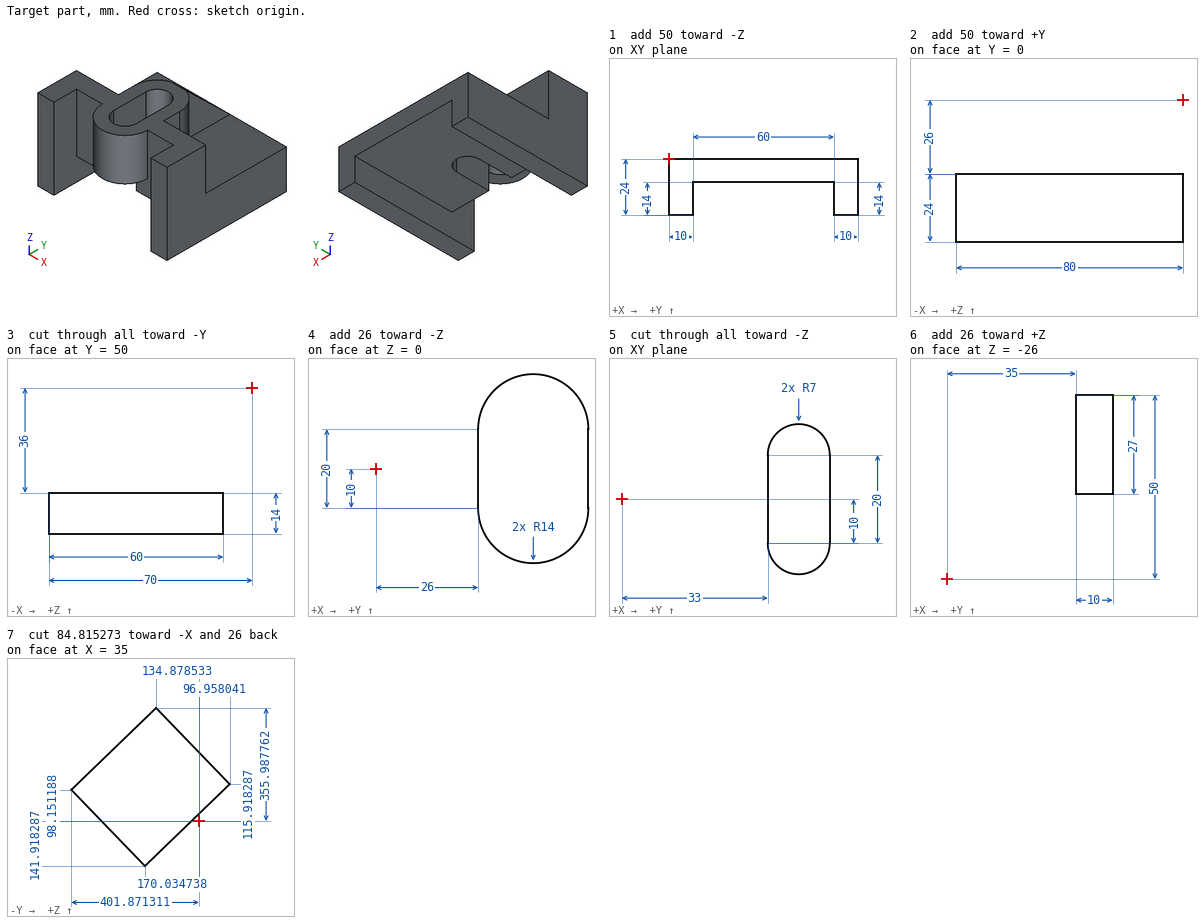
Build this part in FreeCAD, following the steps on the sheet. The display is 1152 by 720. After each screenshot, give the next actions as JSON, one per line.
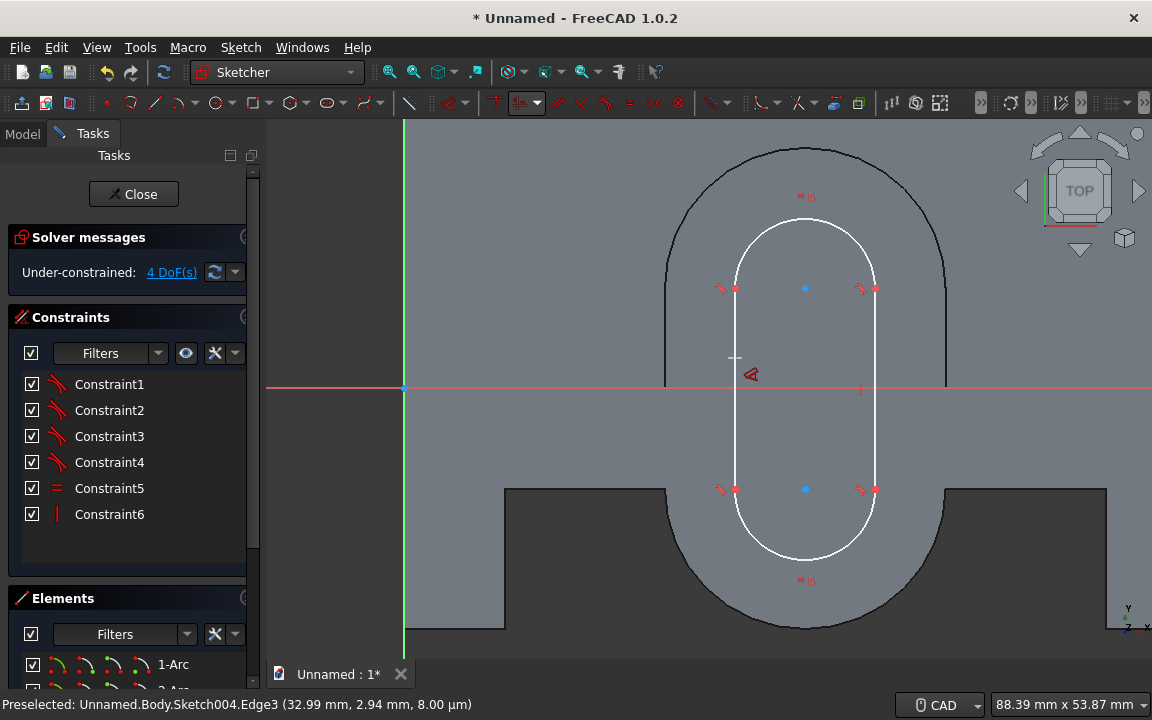
{"action": "left_click", "coordinate": [764, 547]}
{"action": "left_click", "coordinate": [745, 573]}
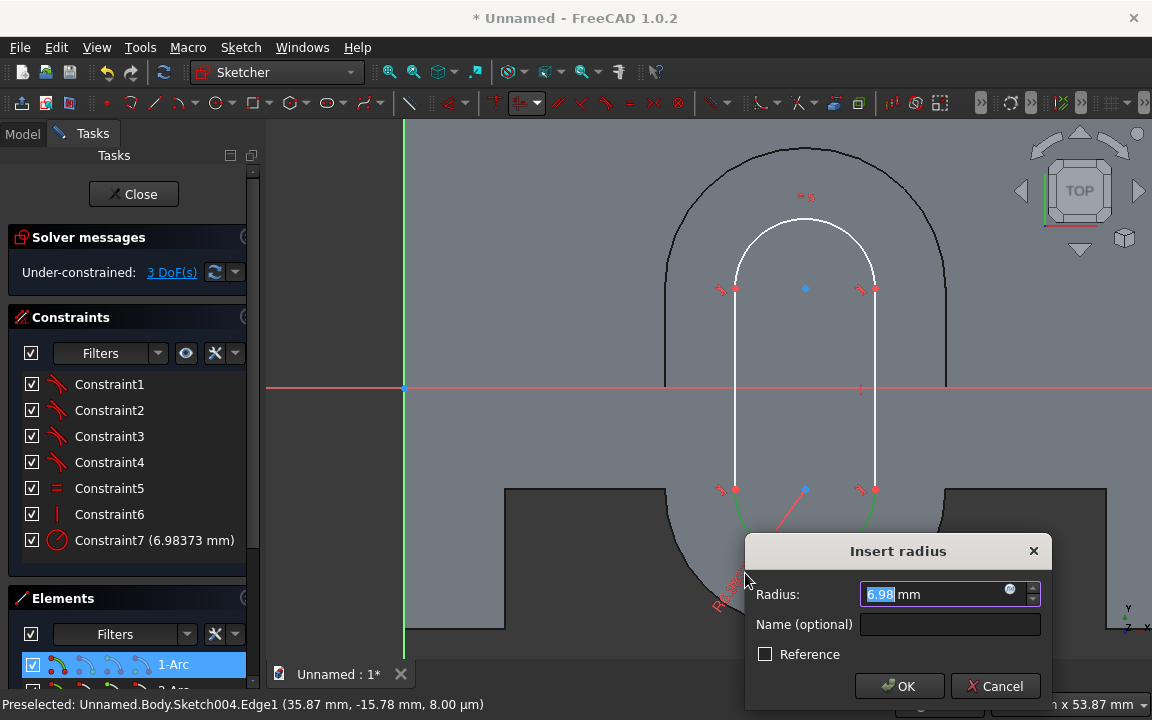
{"action": "type", "text": "7"}
{"action": "key", "text": "Return"}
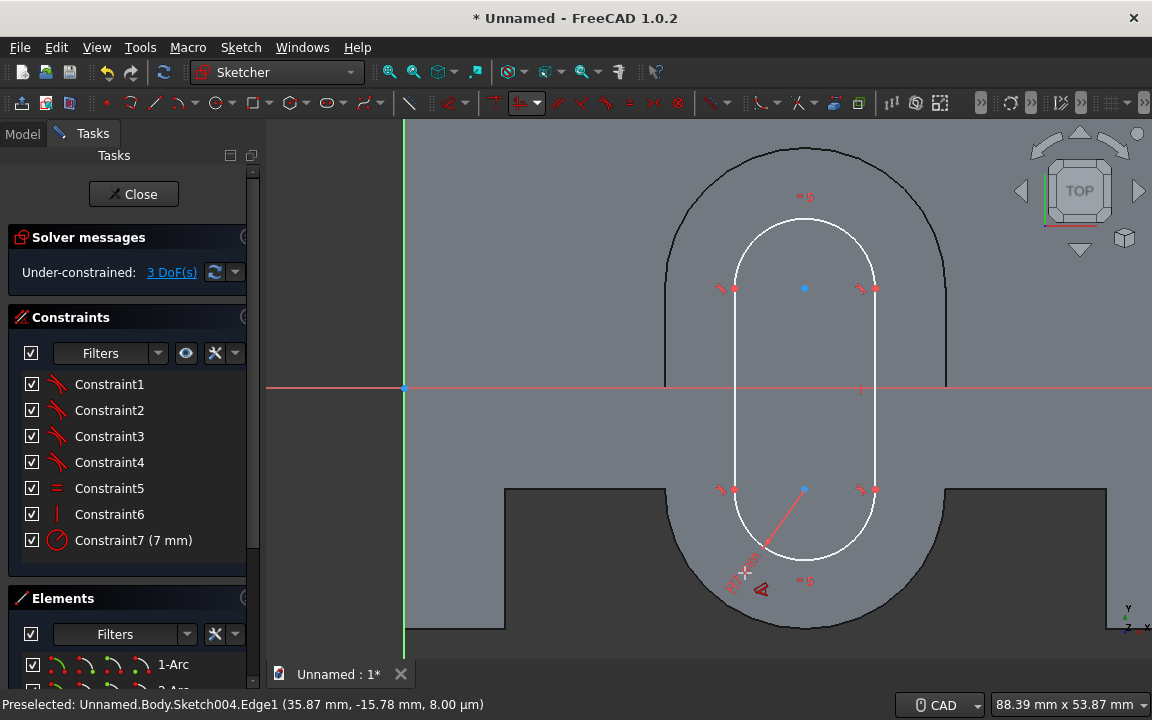
{"action": "left_click", "coordinate": [735, 430]}
{"action": "left_click", "coordinate": [769, 343]}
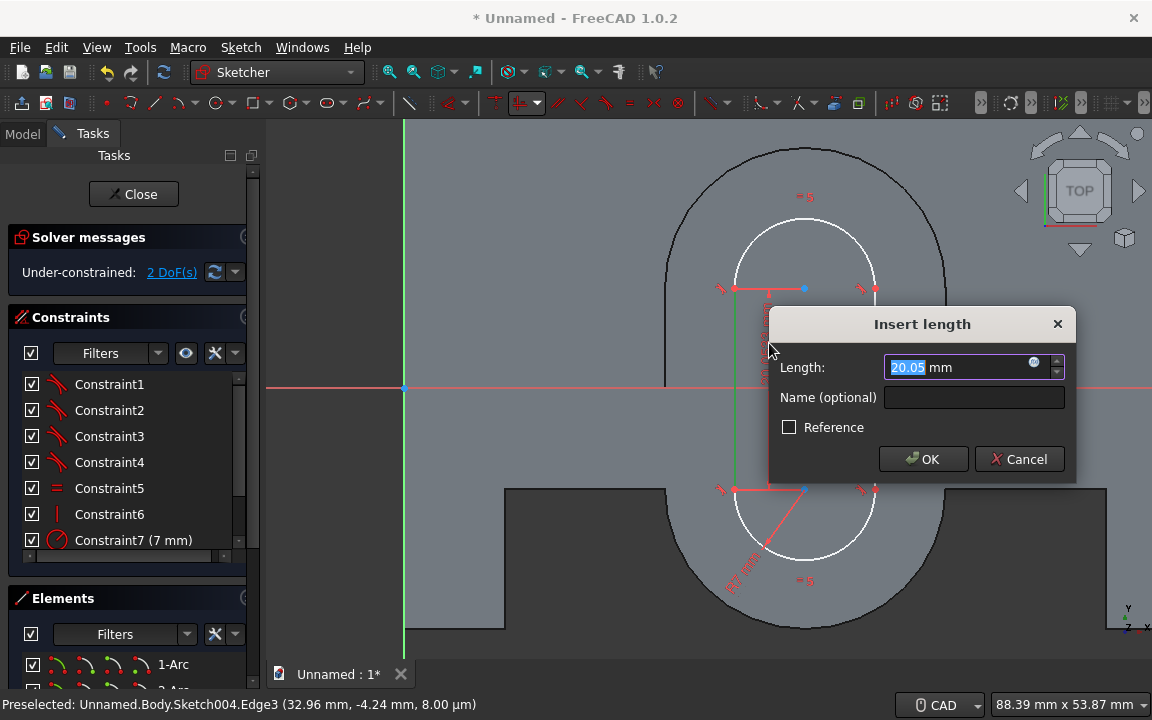
{"action": "type", "text": "20"}
{"action": "key", "text": "Return"}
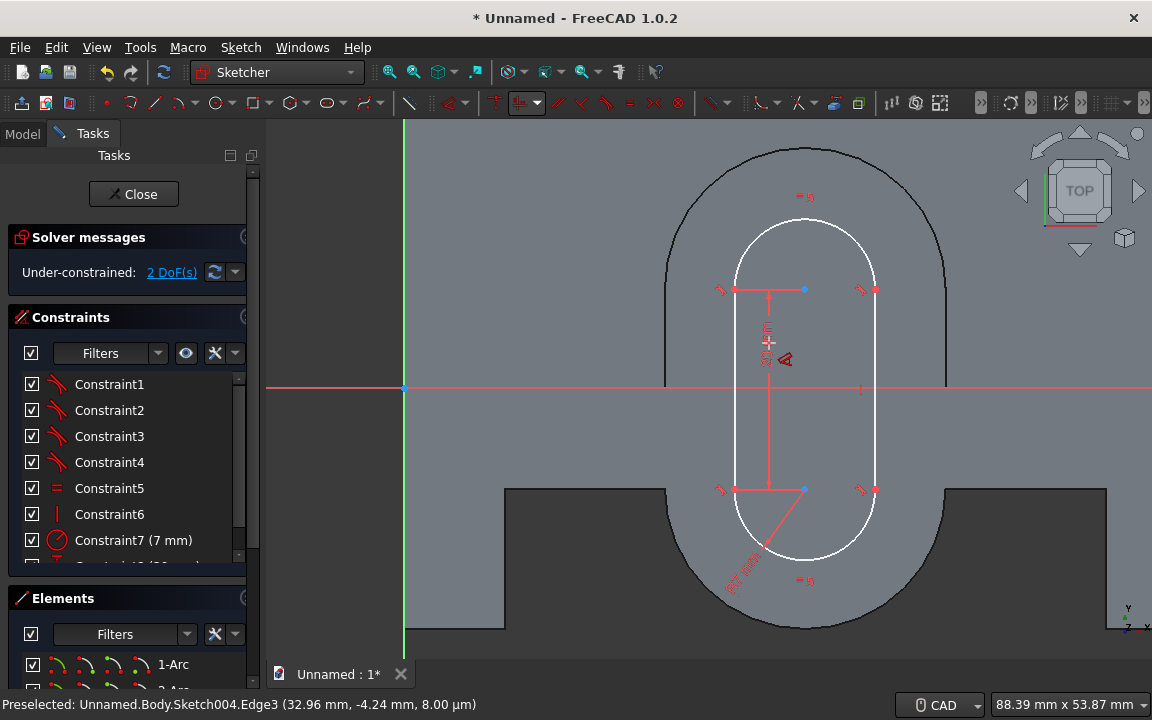
{"action": "left_click", "coordinate": [735, 490]}
{"action": "left_click", "coordinate": [569, 524]}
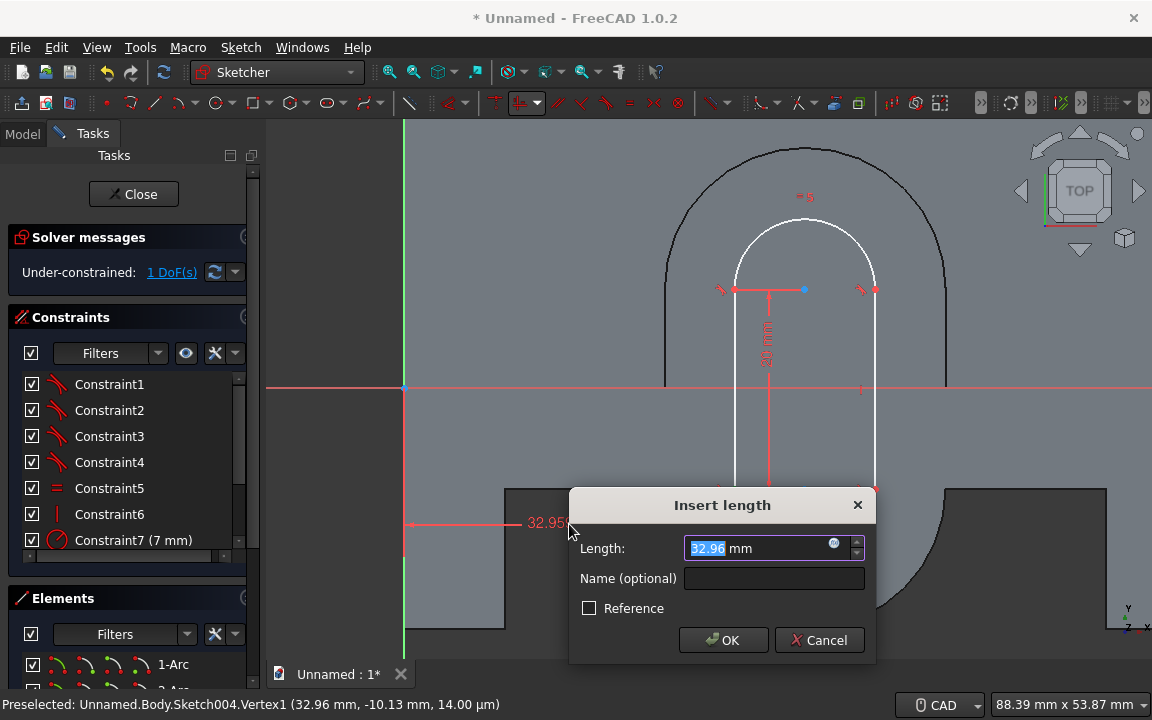
{"action": "type", "text": "33"}
{"action": "key", "text": "Return"}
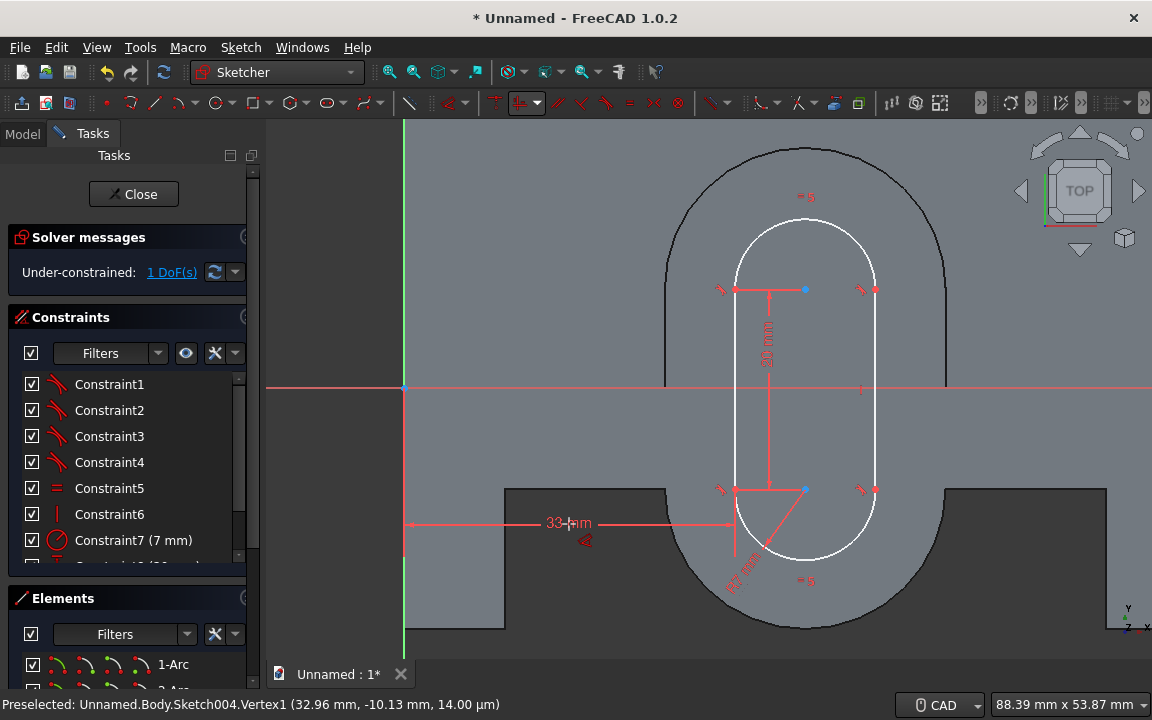
{"action": "left_click", "coordinate": [735, 490]}
{"action": "left_click", "coordinate": [370, 439]}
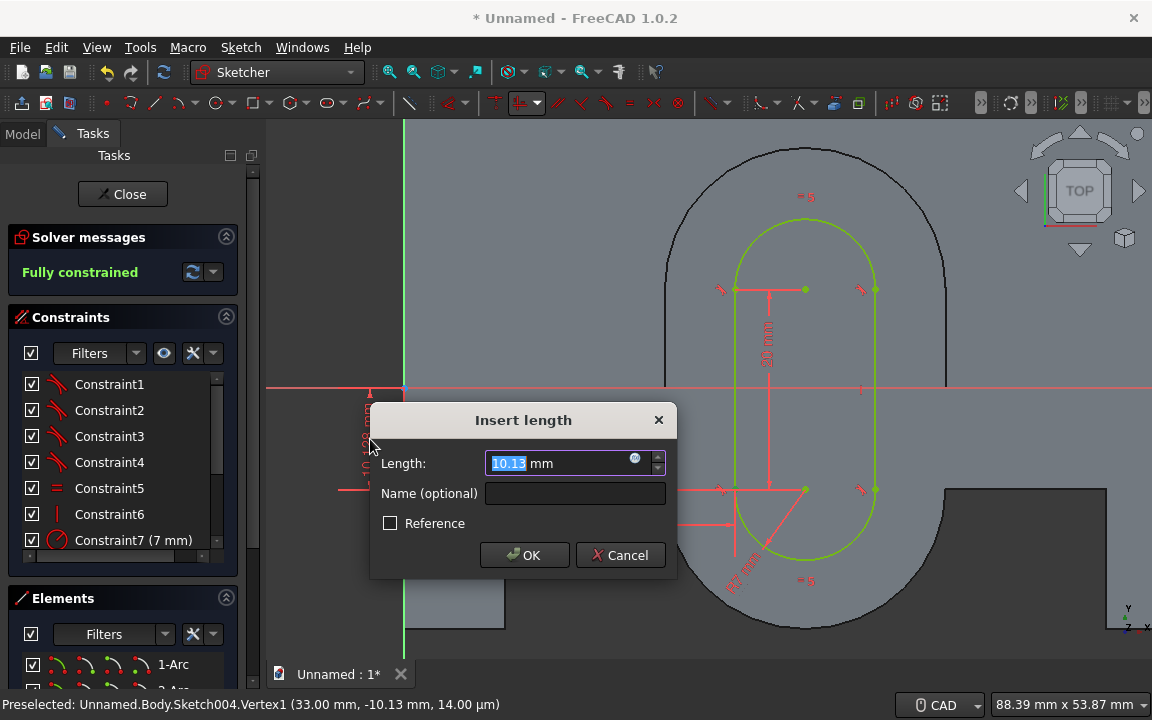
{"action": "type", "text": "10"}
{"action": "key", "text": "Return"}
{"action": "key", "text": "Escape"}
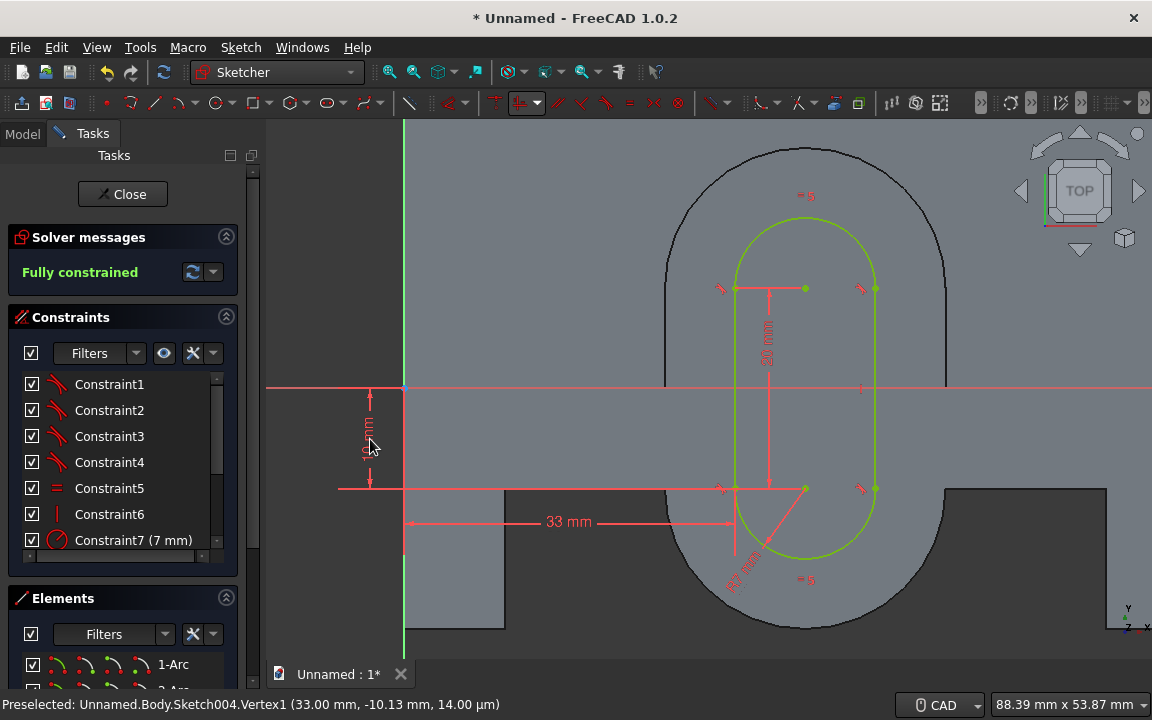
{"action": "left_click", "coordinate": [123, 194]}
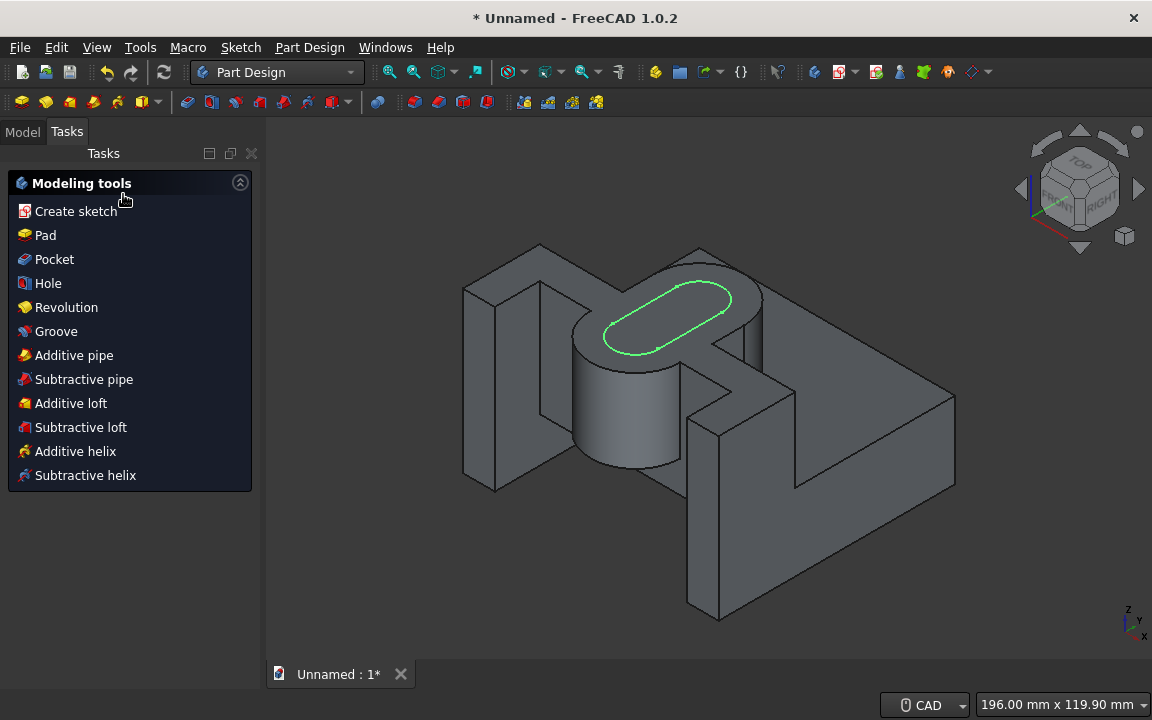
{"action": "left_click", "coordinate": [188, 102]}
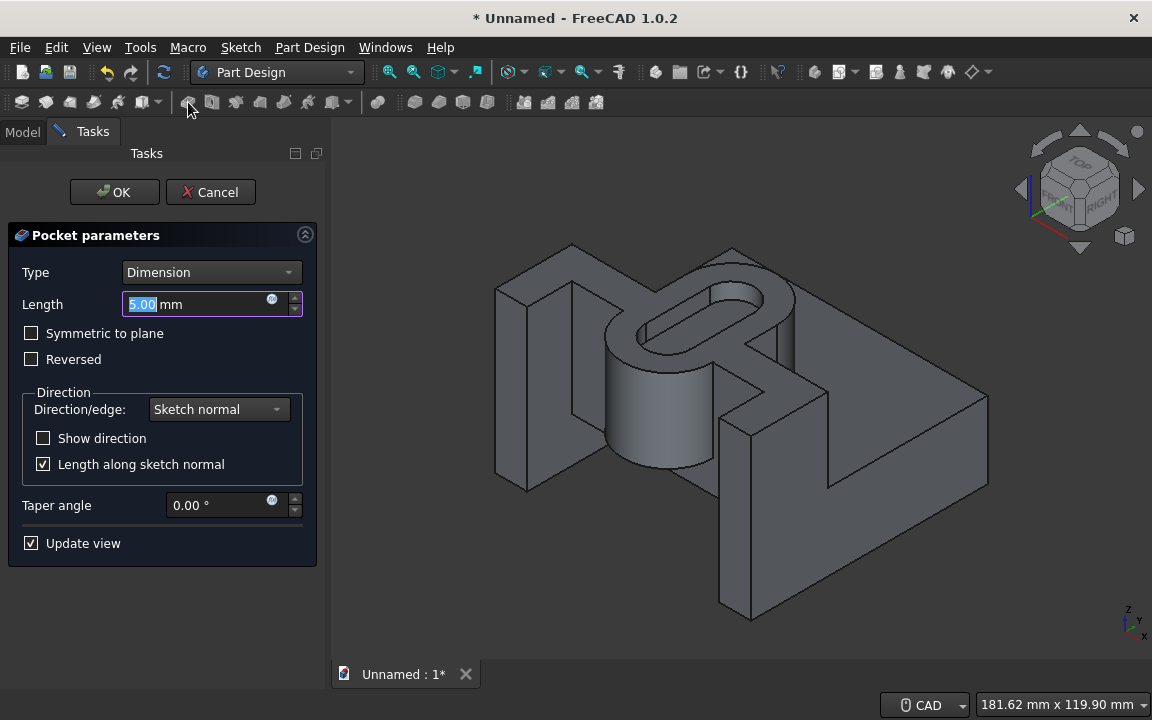
{"action": "left_click", "coordinate": [212, 272]}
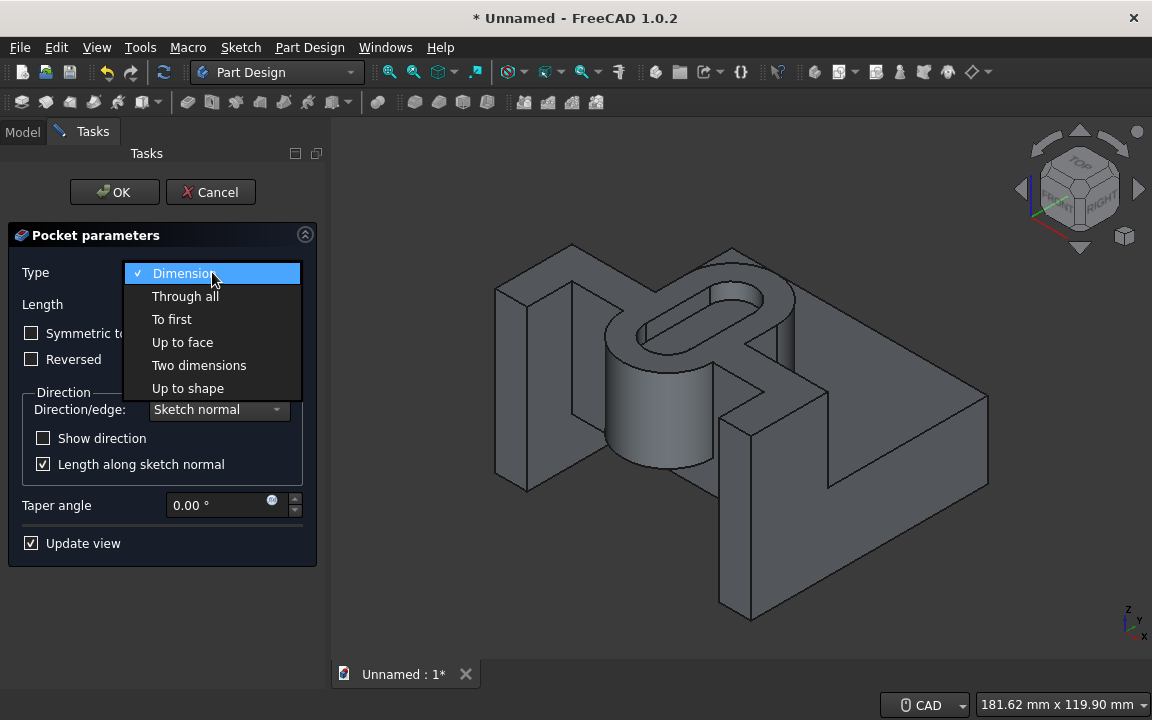
{"action": "left_click", "coordinate": [212, 296]}